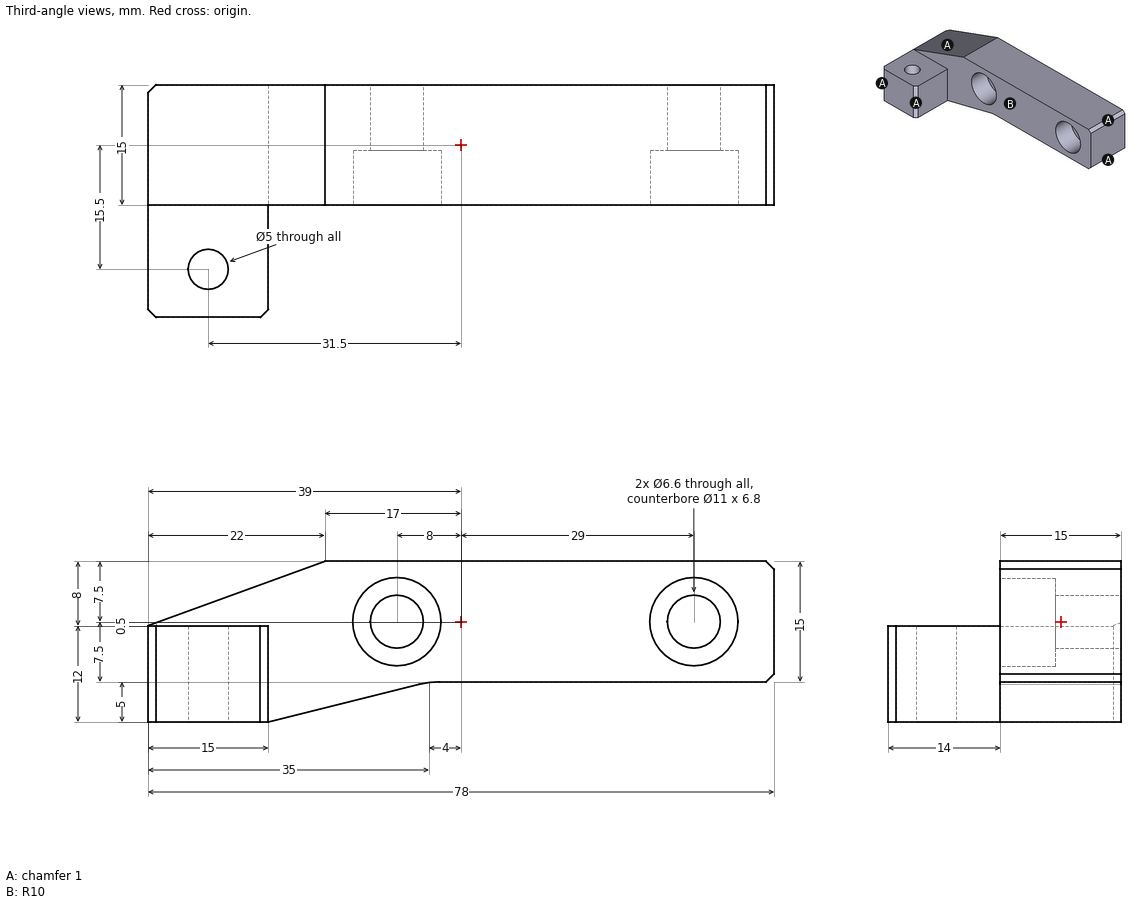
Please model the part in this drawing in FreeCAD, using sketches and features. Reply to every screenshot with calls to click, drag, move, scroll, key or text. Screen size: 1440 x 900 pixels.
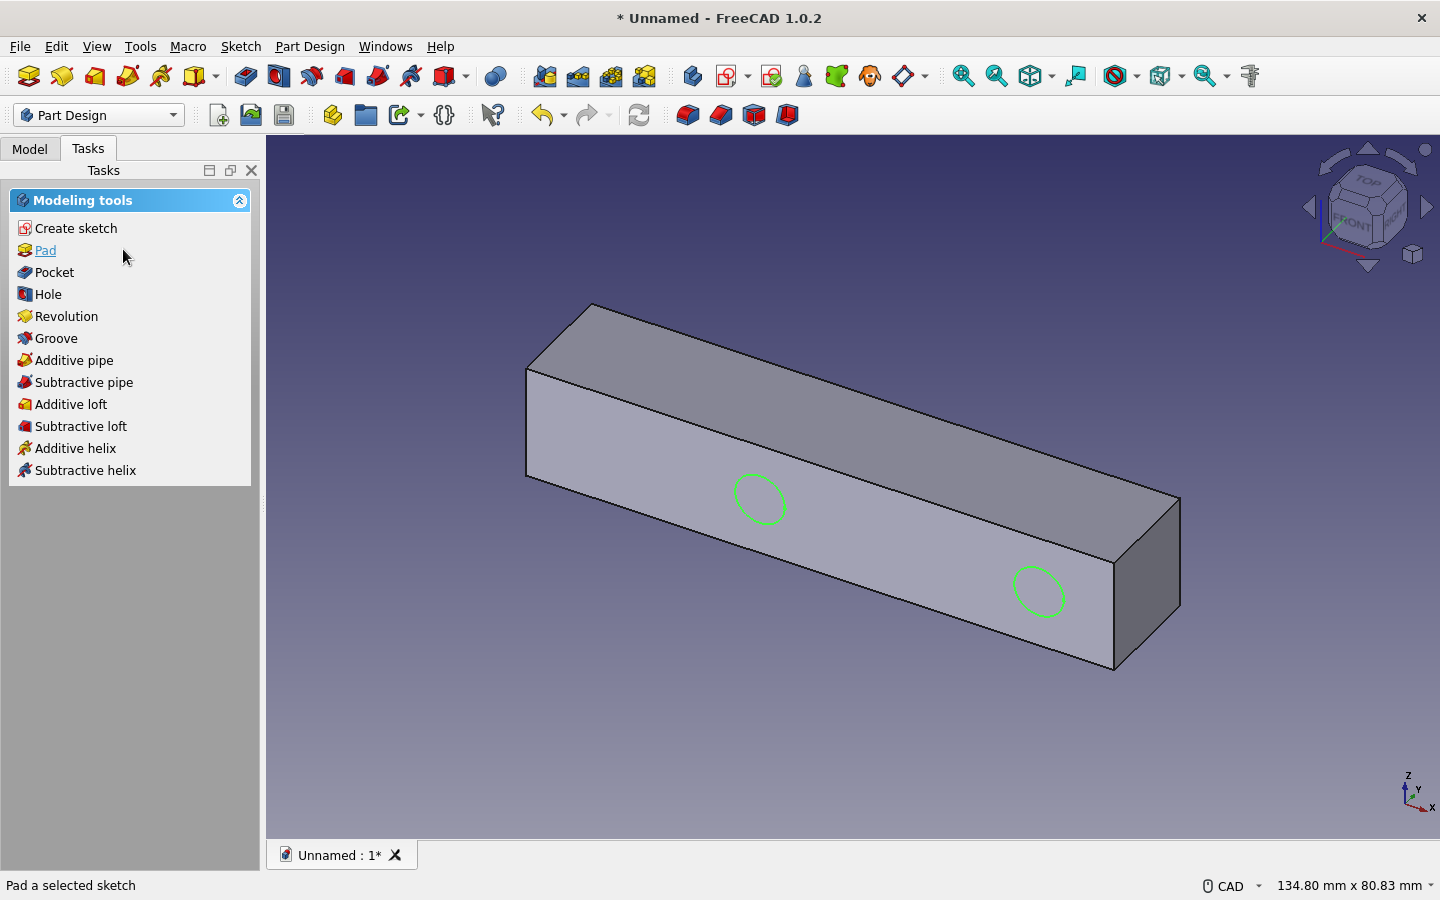
click(279, 76)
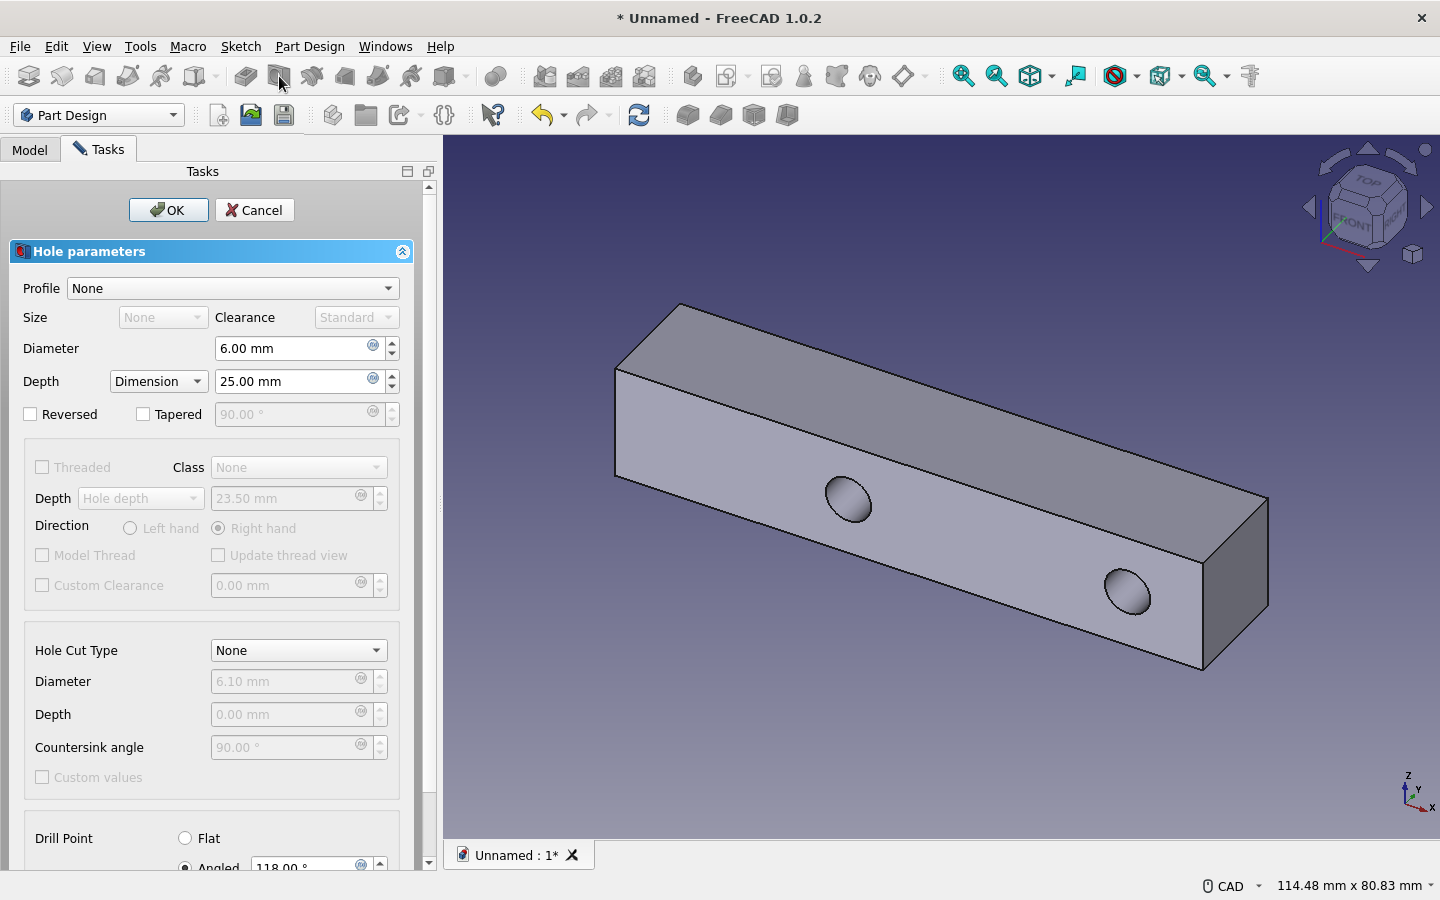
triple_click(300, 348)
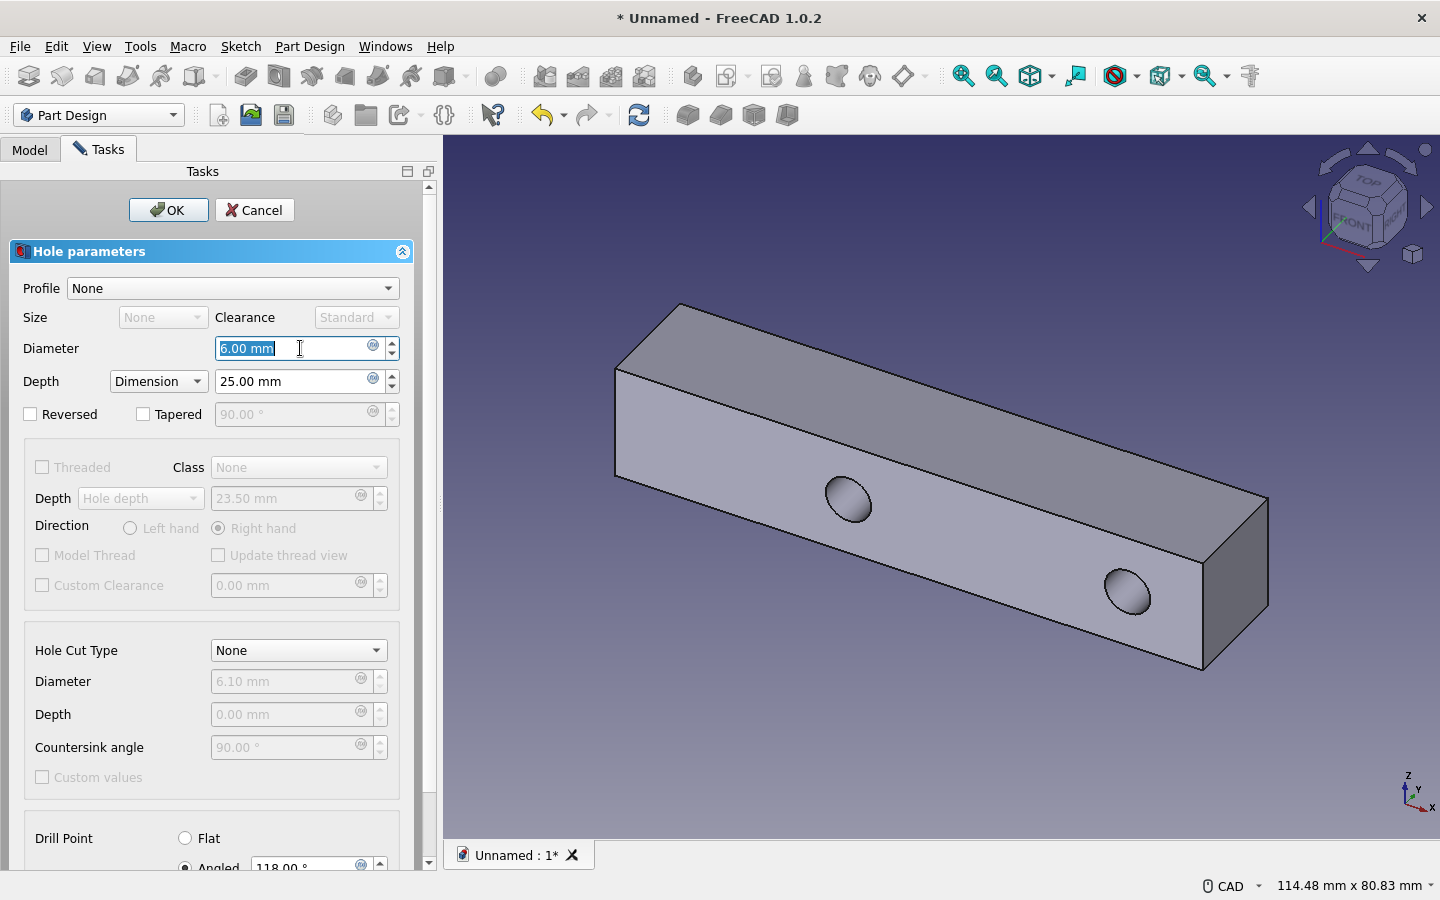
text(6.6)
key(Tab)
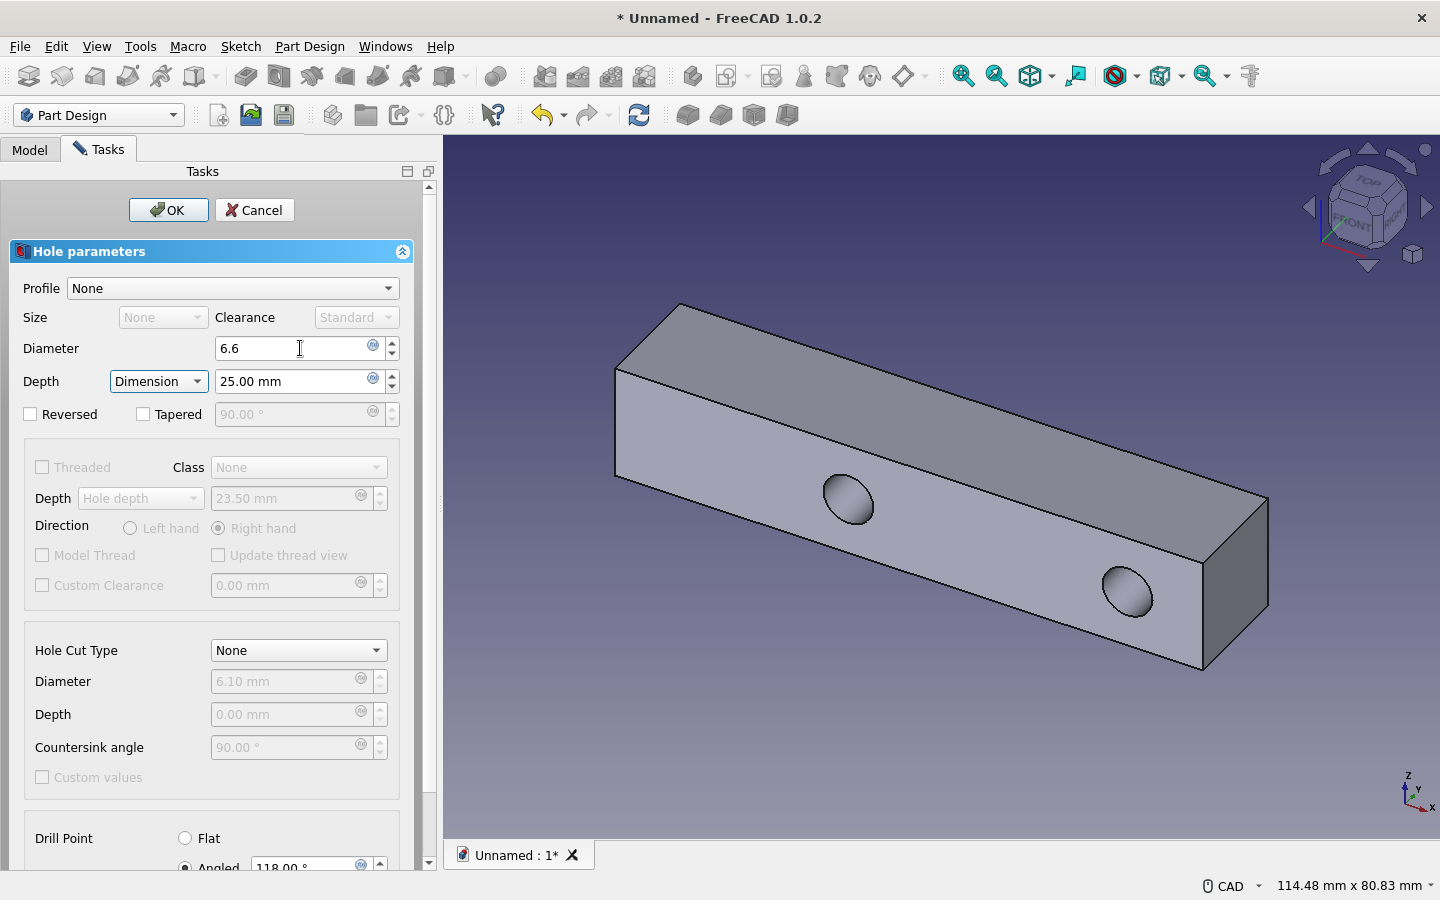
click(160, 382)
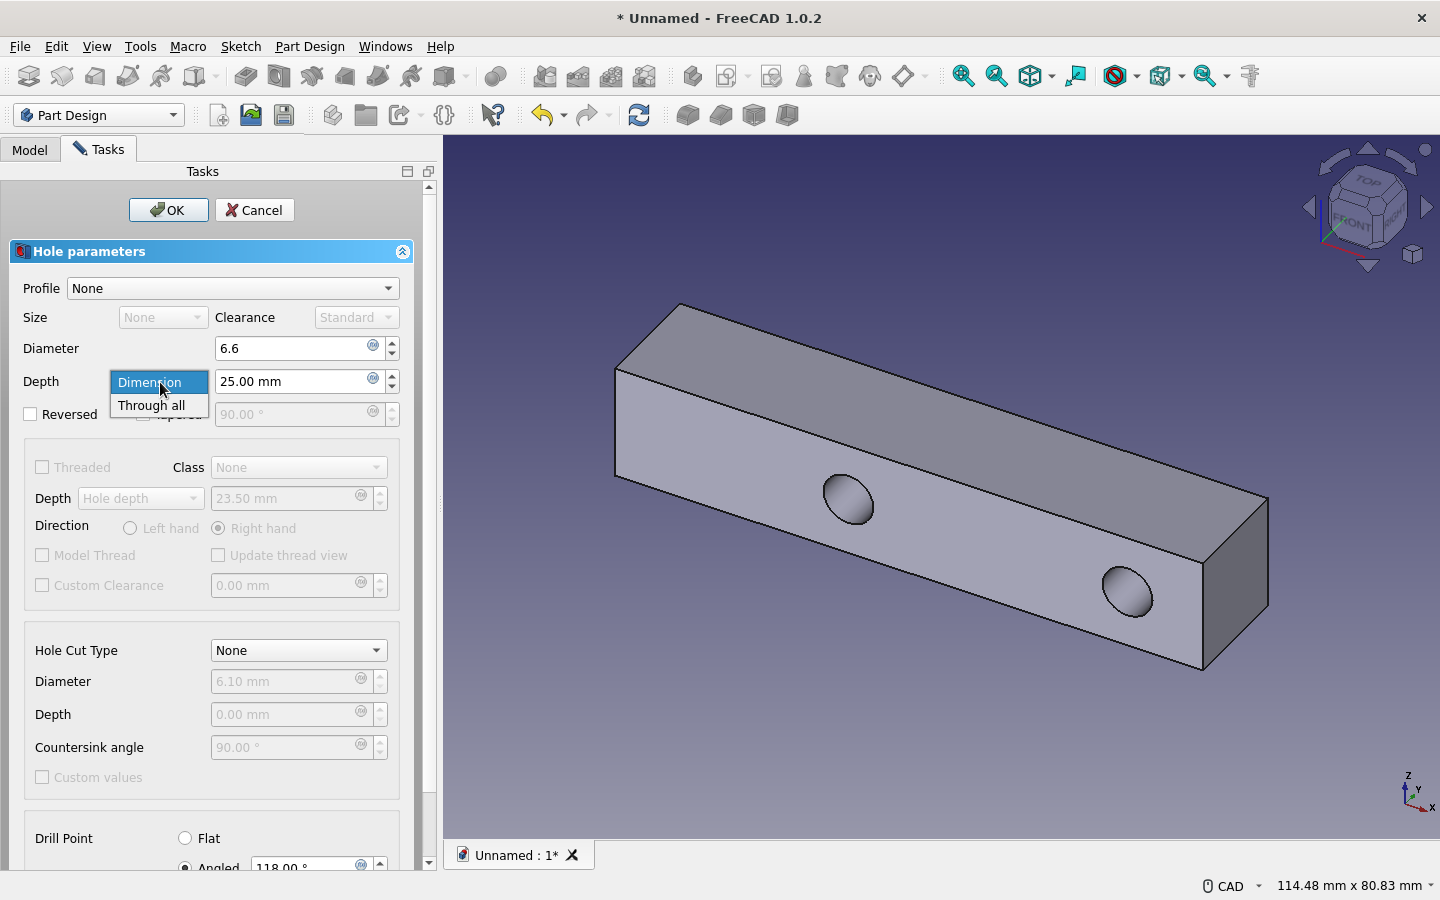
click(158, 406)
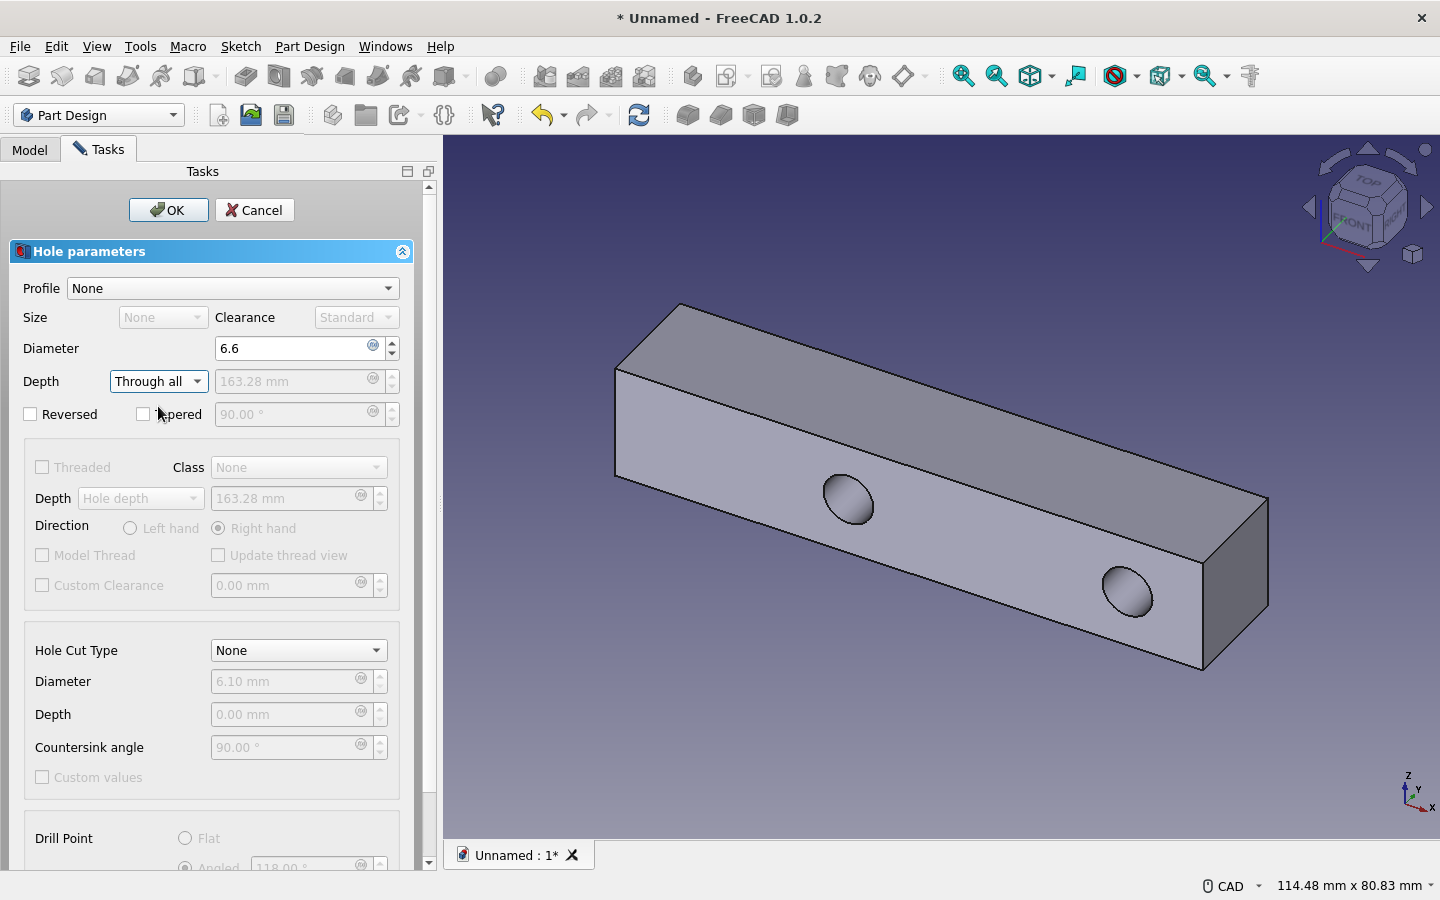
click(300, 650)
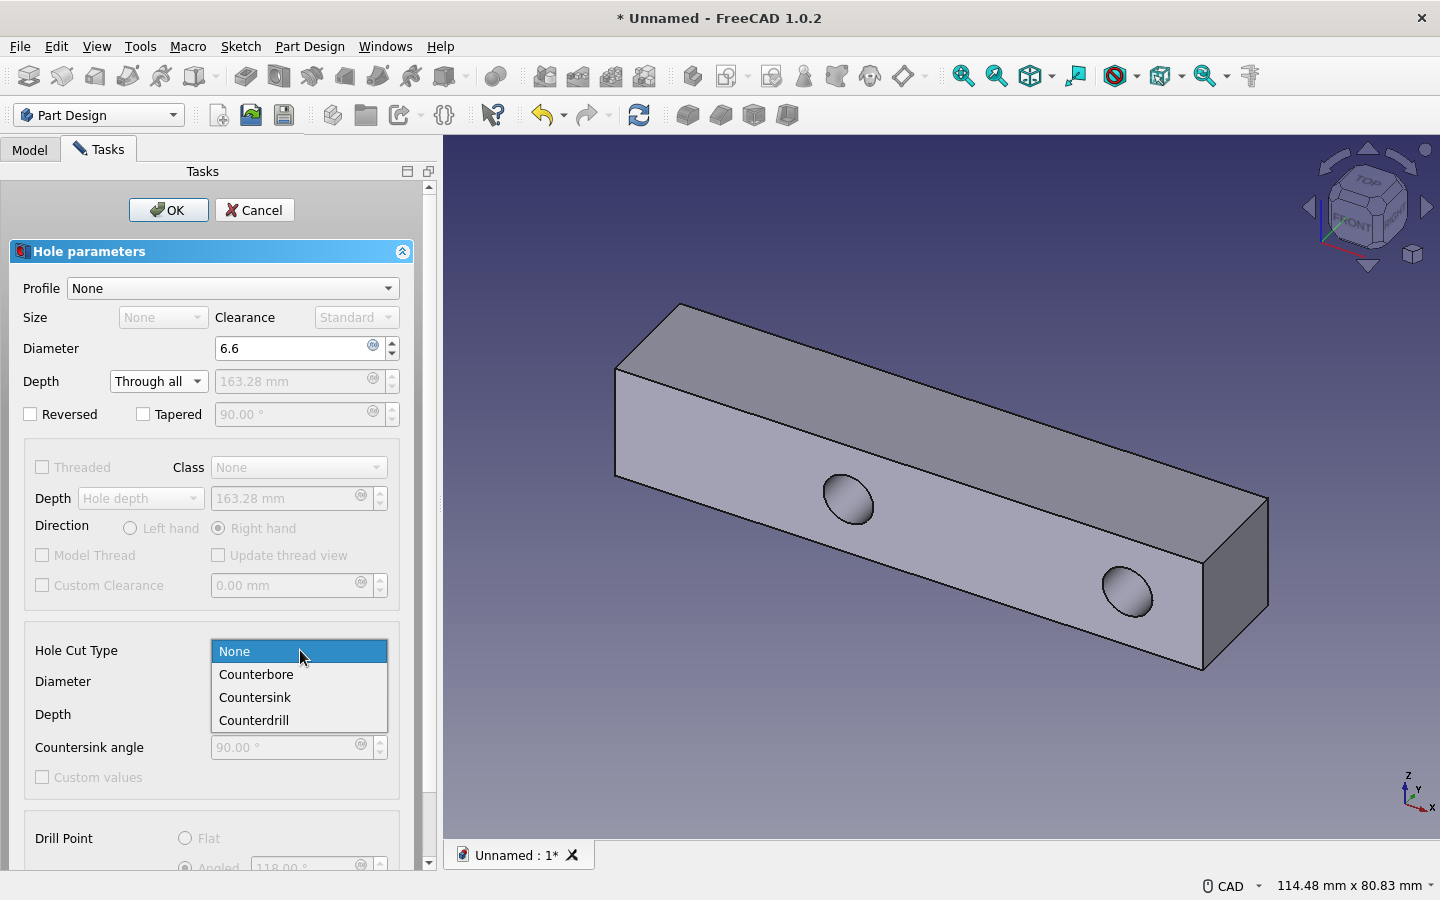
click(298, 674)